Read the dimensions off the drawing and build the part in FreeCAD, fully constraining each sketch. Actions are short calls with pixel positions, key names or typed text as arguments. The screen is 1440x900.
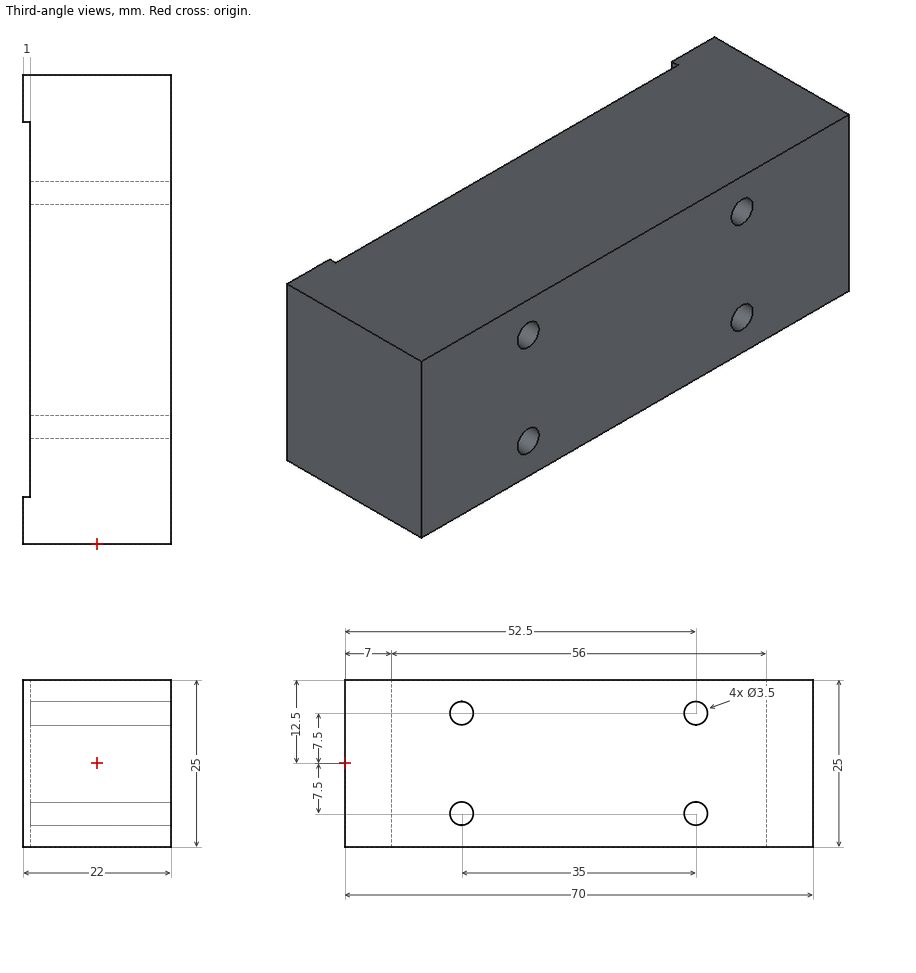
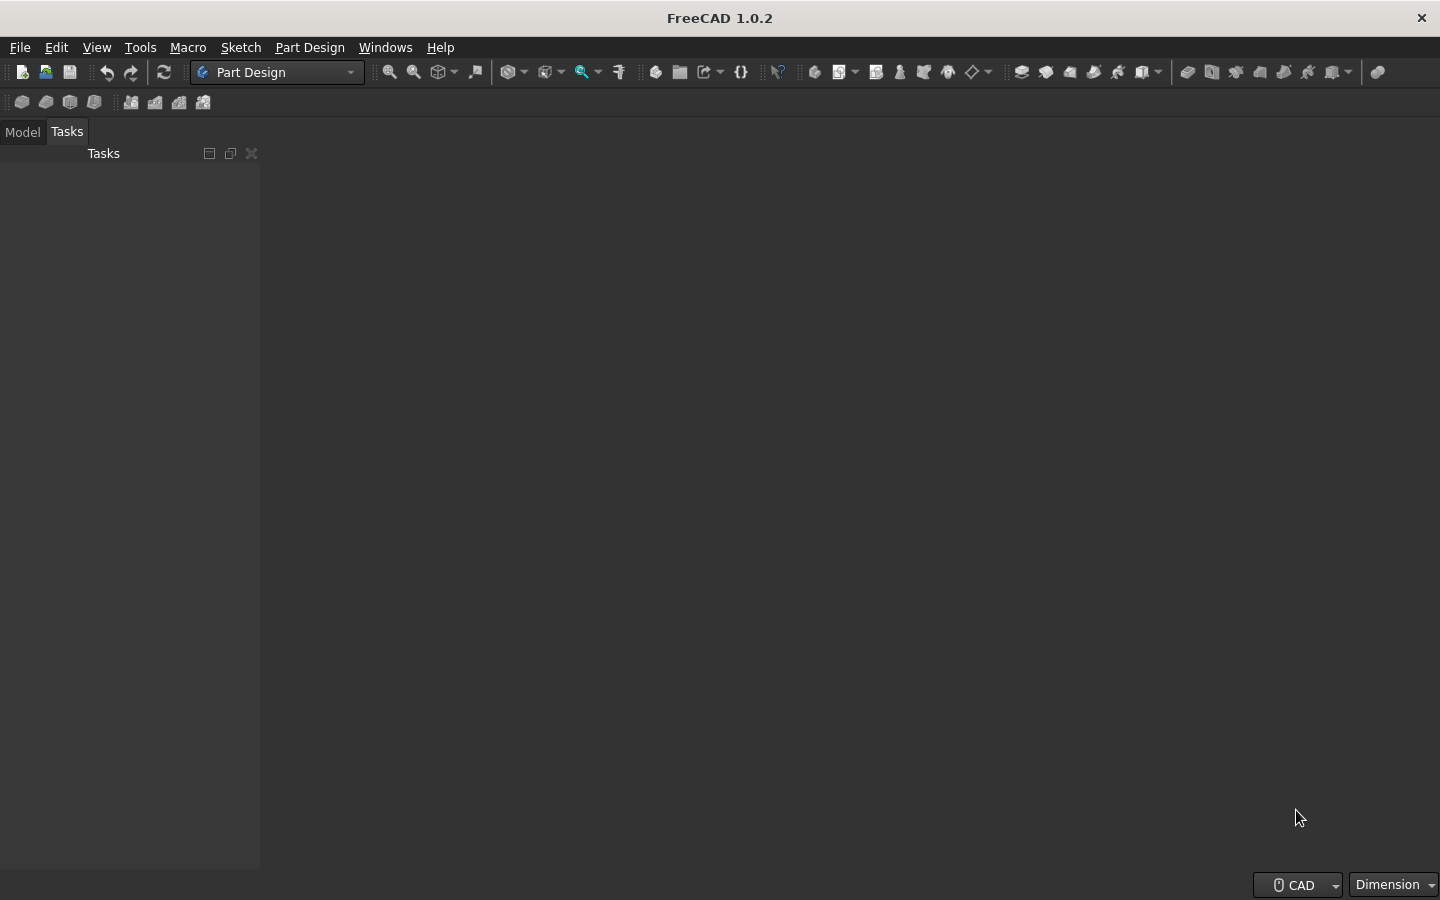
click(22, 72)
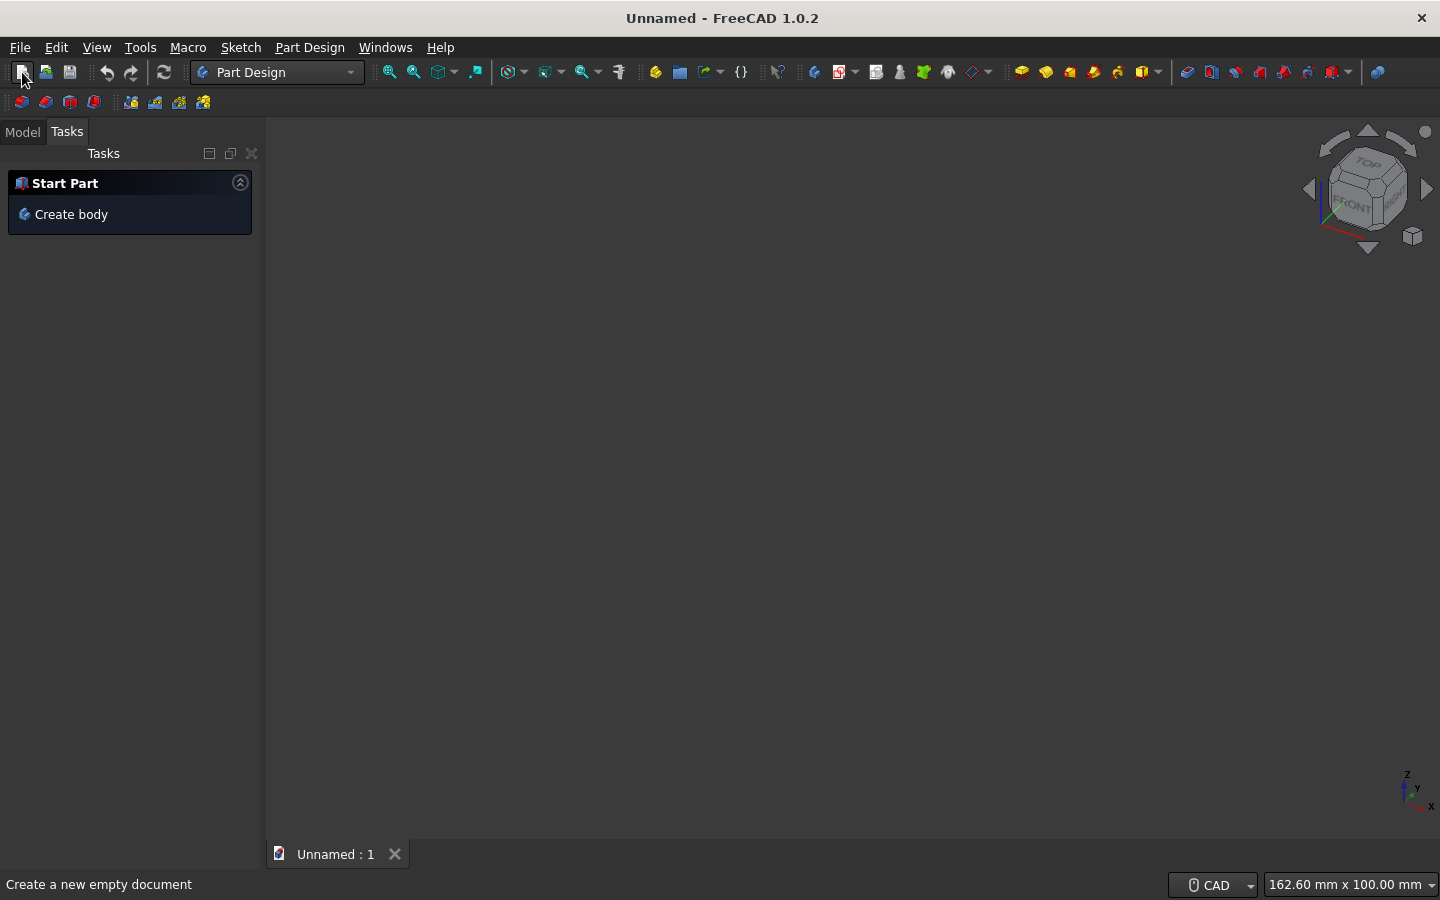
click(840, 72)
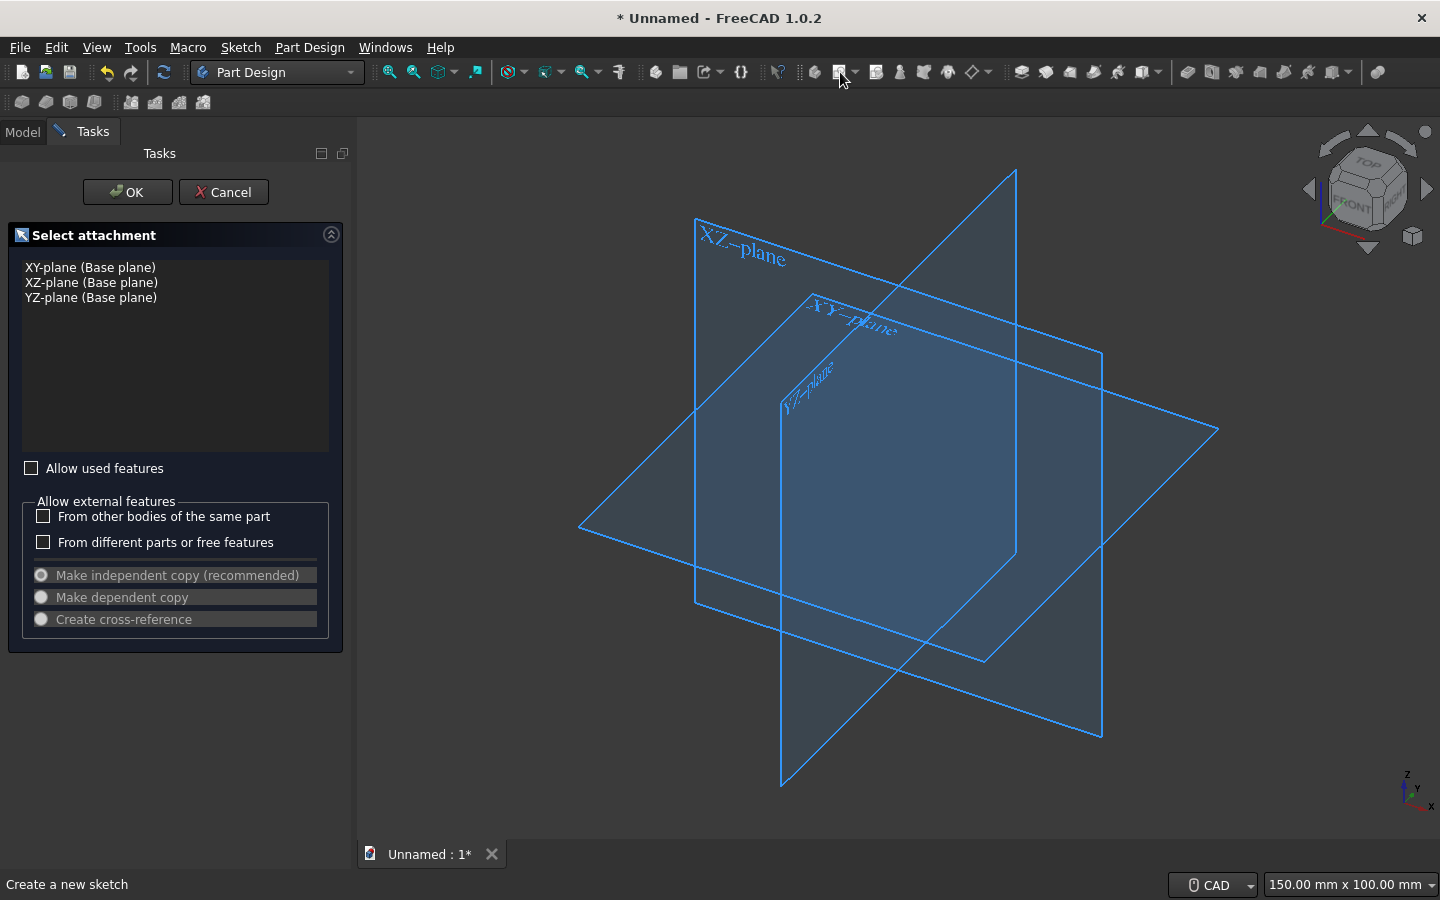
click(82, 282)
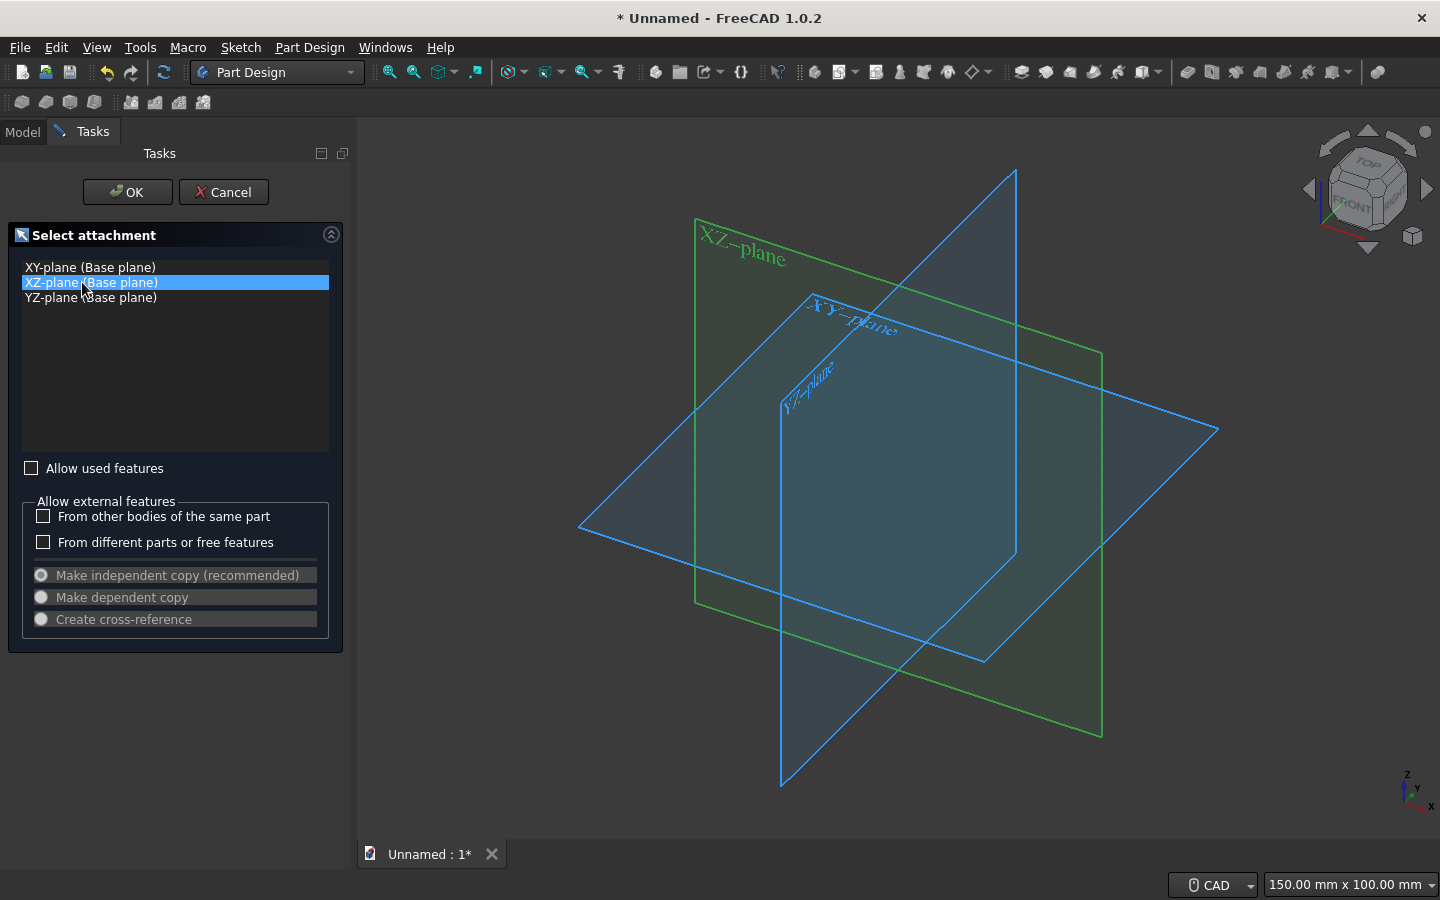
click(128, 192)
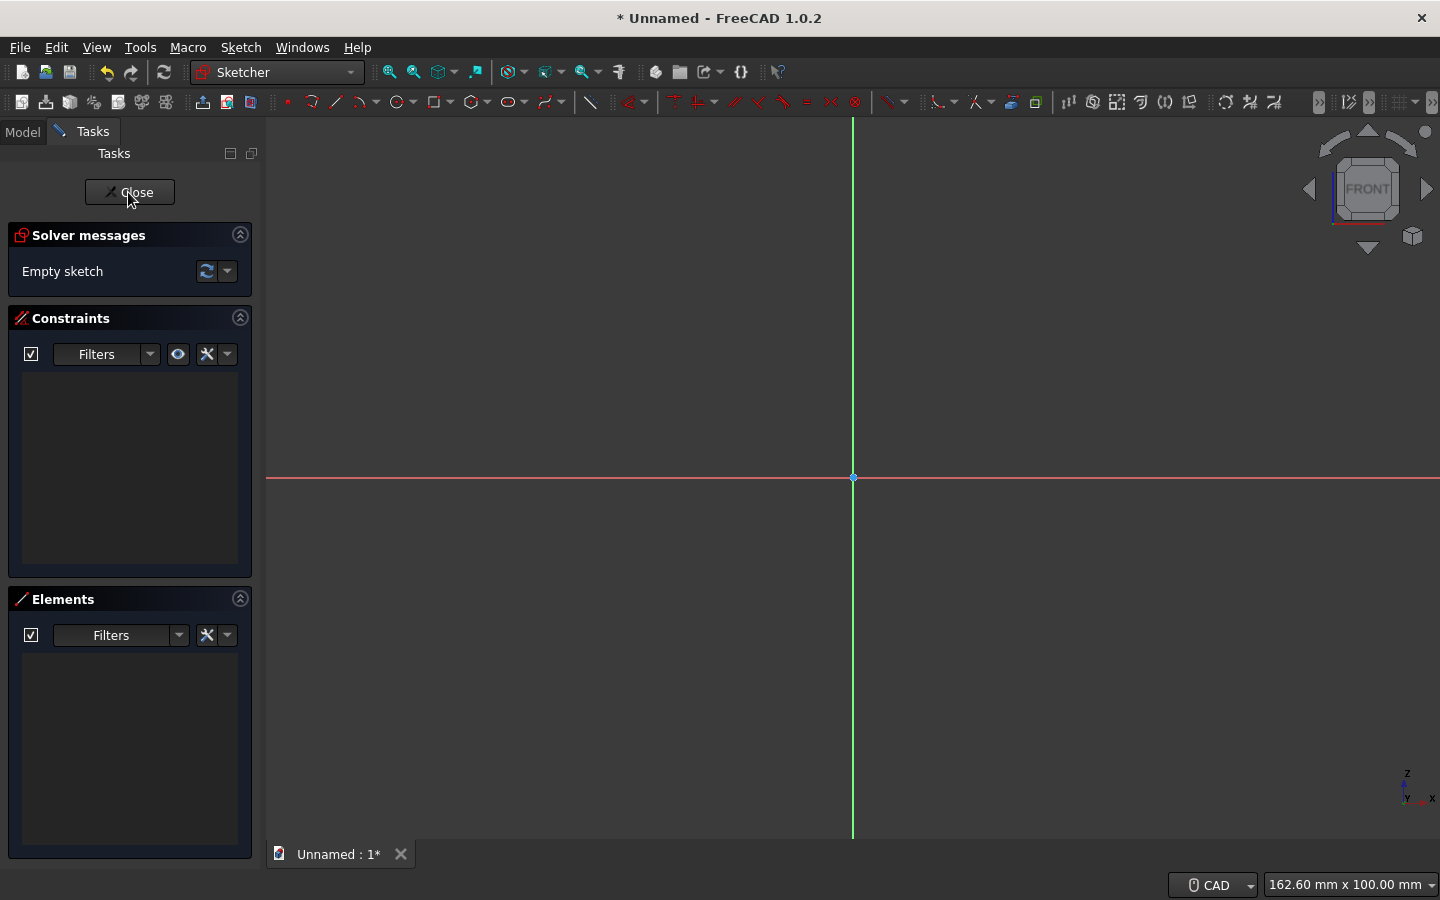
scroll(893, 478, up, 5)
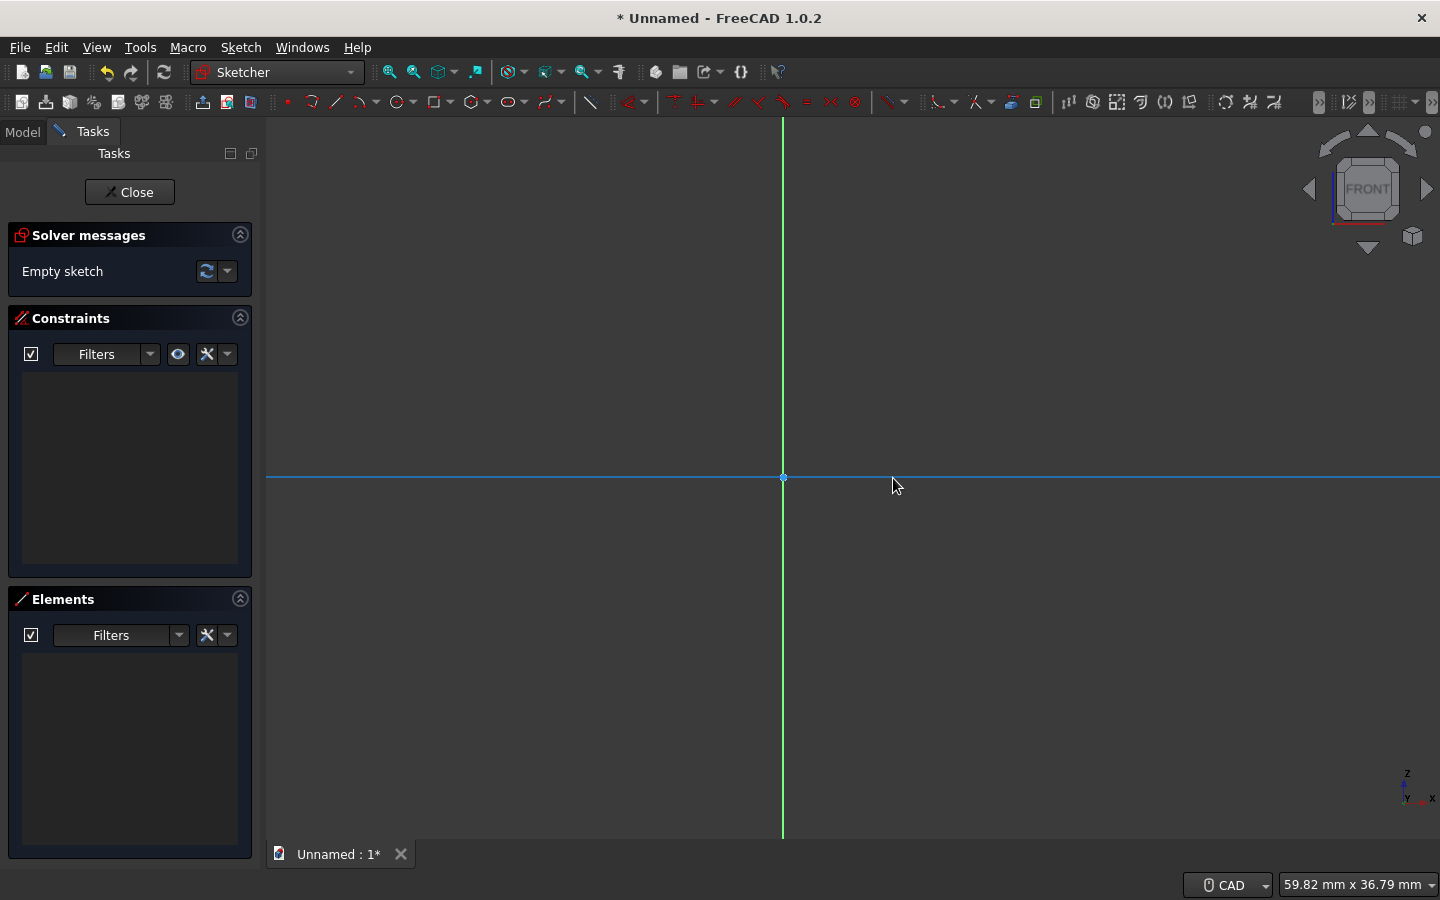
key(g)
key(v)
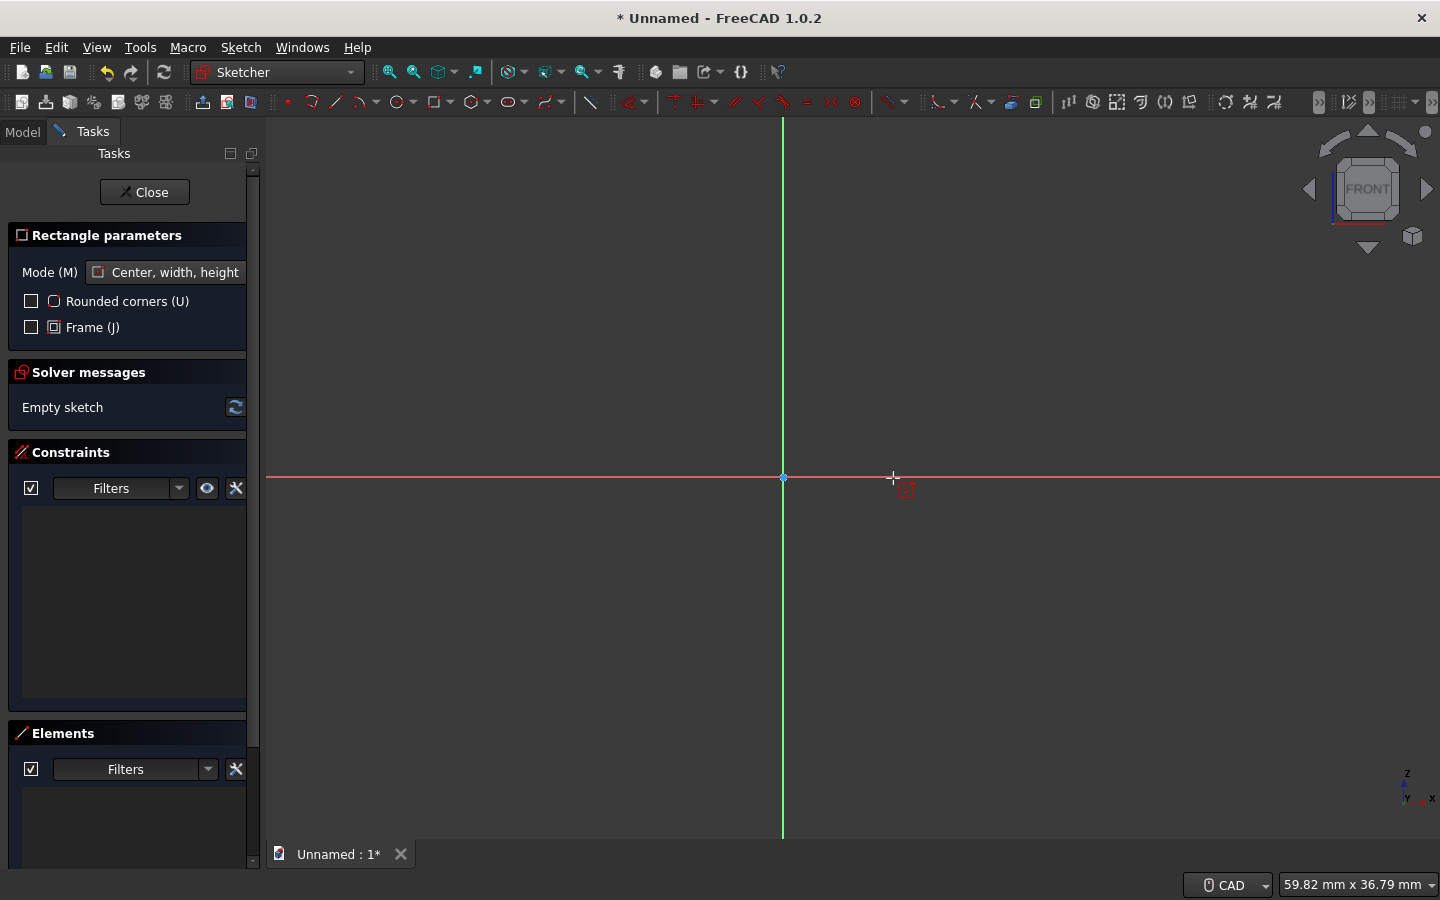
click(783, 477)
click(999, 232)
key(Escape)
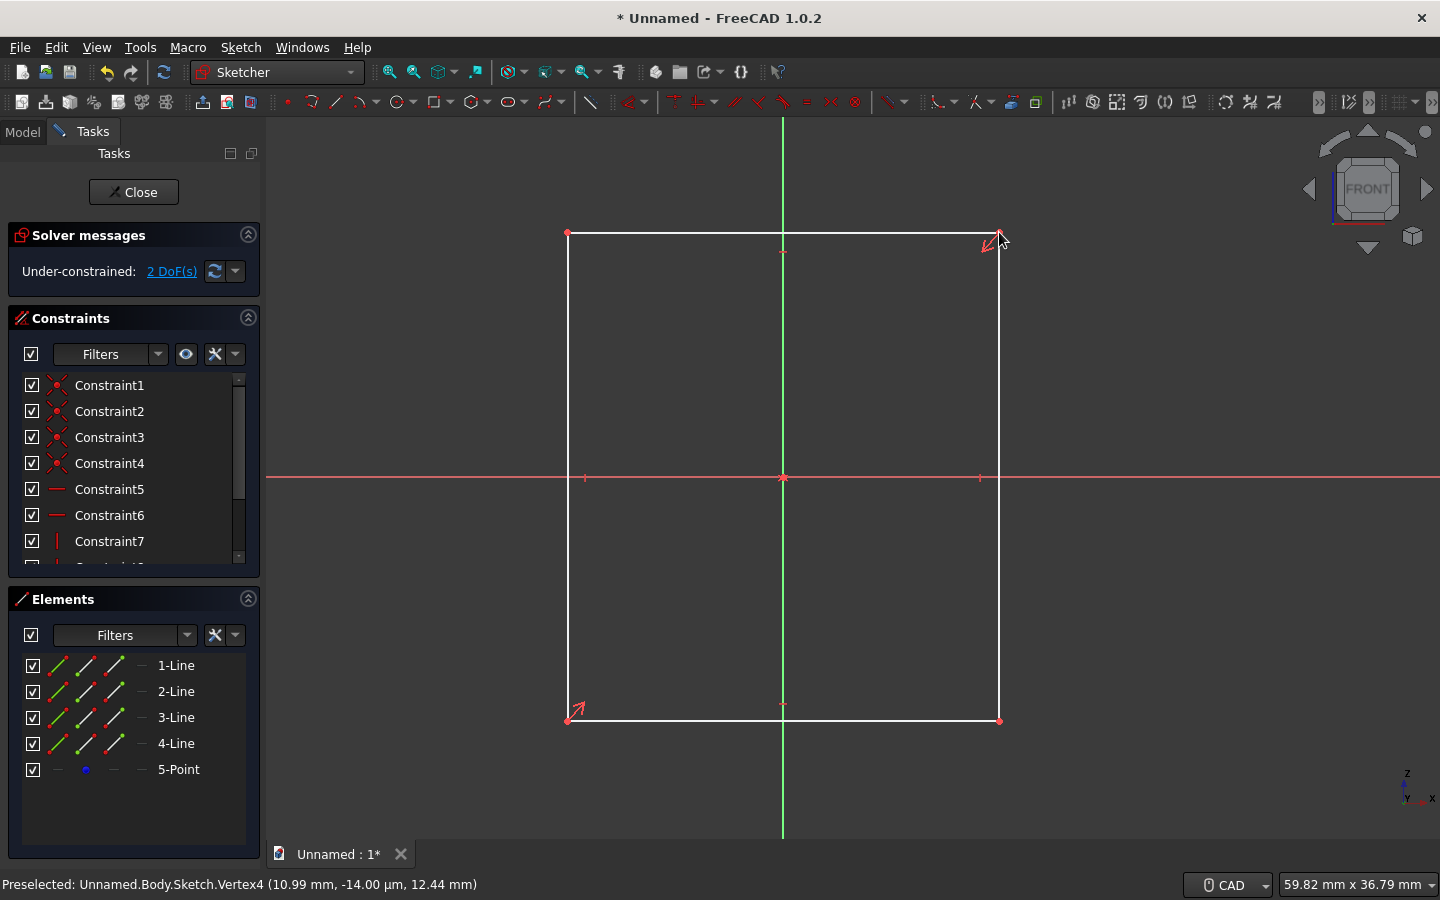
click(697, 721)